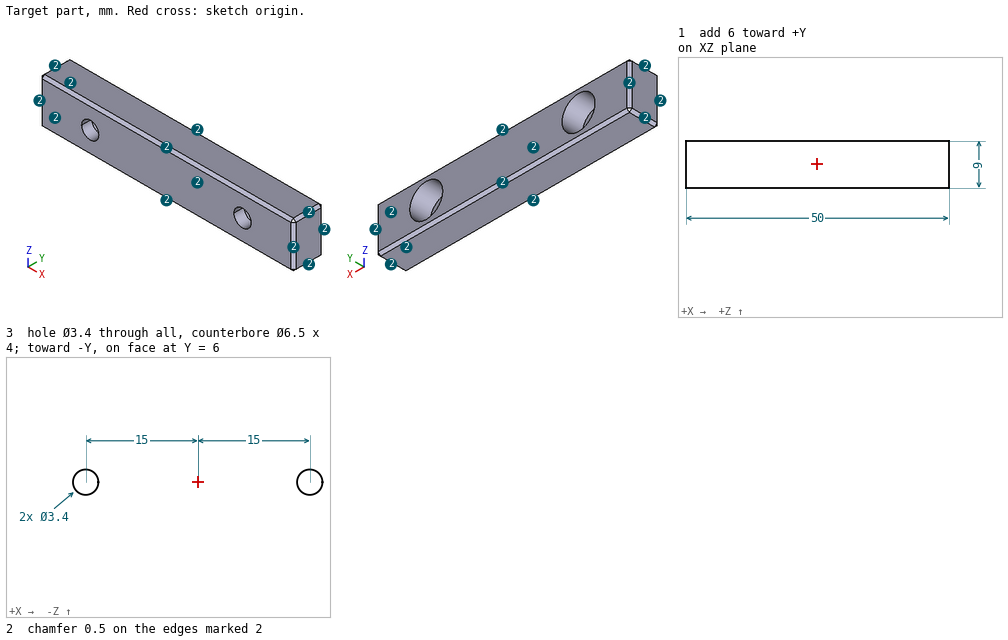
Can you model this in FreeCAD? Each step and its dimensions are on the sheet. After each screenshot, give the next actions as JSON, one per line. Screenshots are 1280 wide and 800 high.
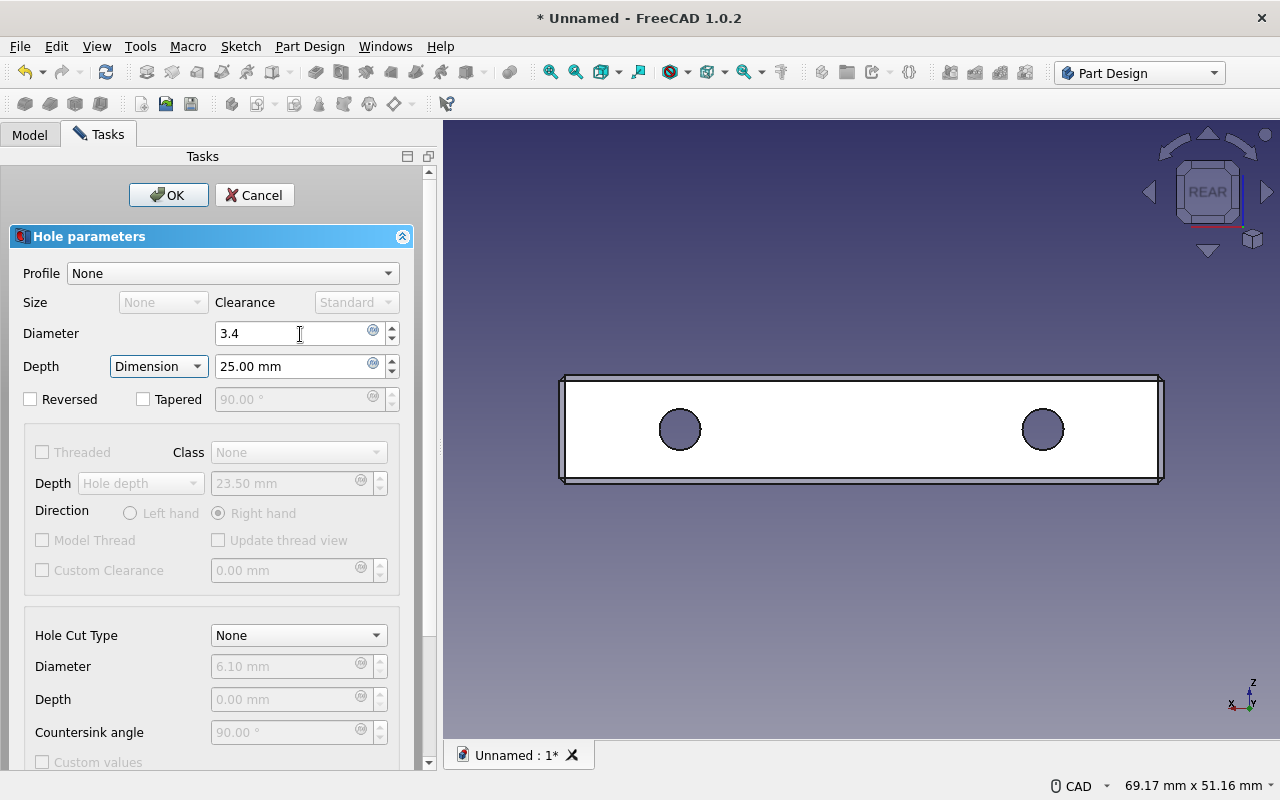
{"action": "left_click", "coordinate": [160, 366]}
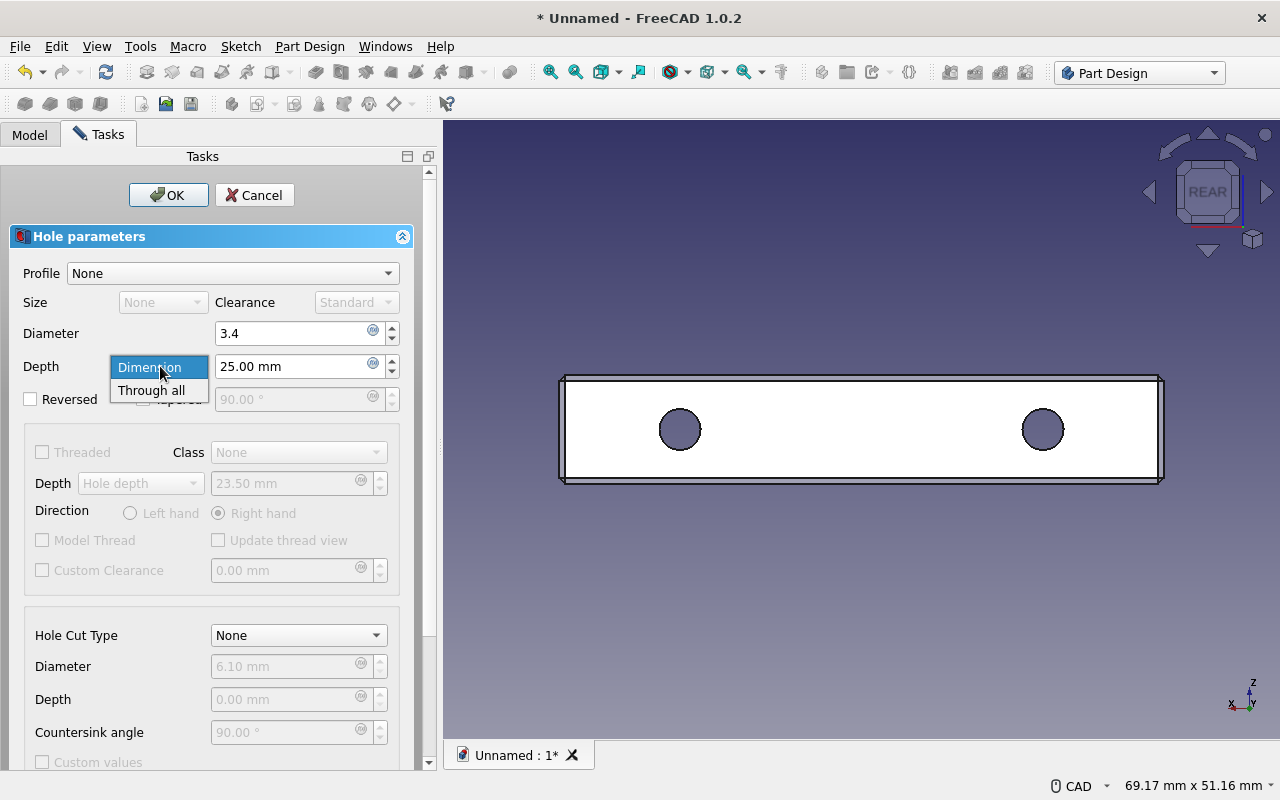
{"action": "left_click", "coordinate": [158, 390]}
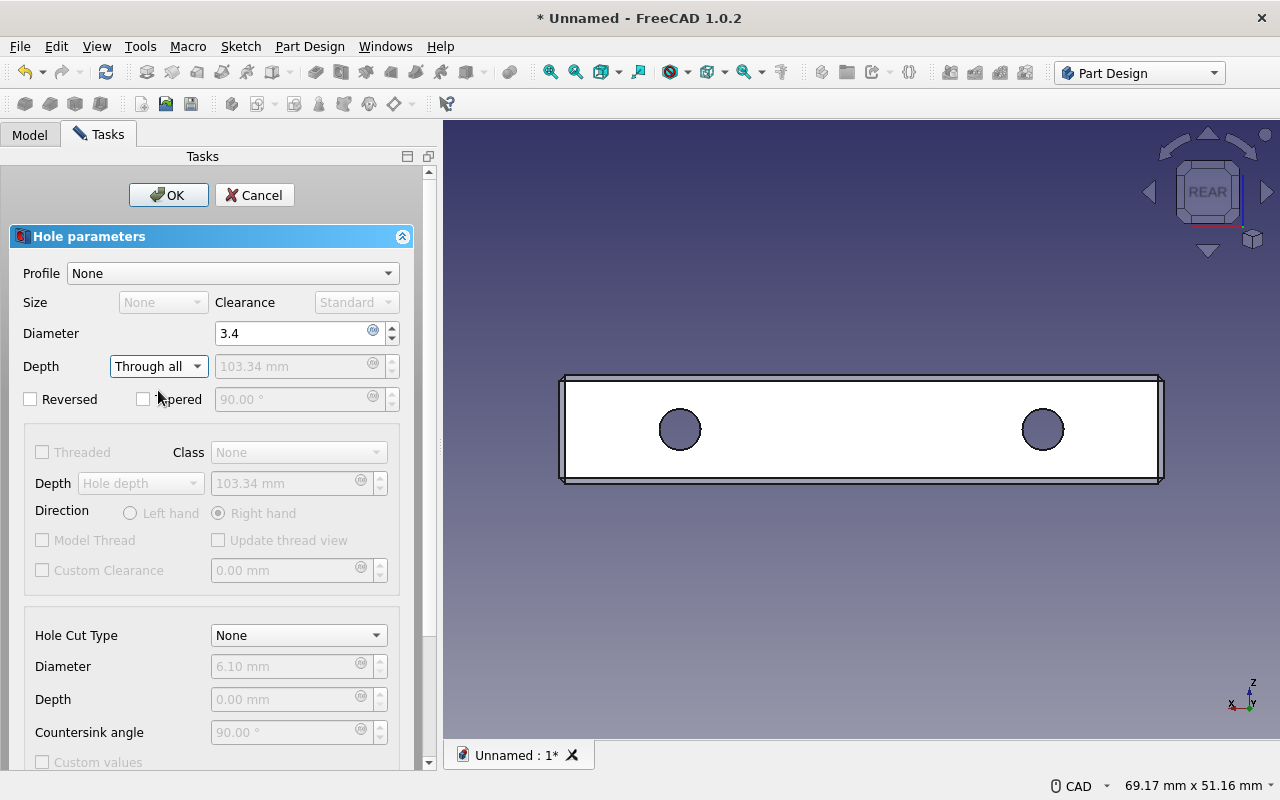
{"action": "left_click", "coordinate": [300, 636]}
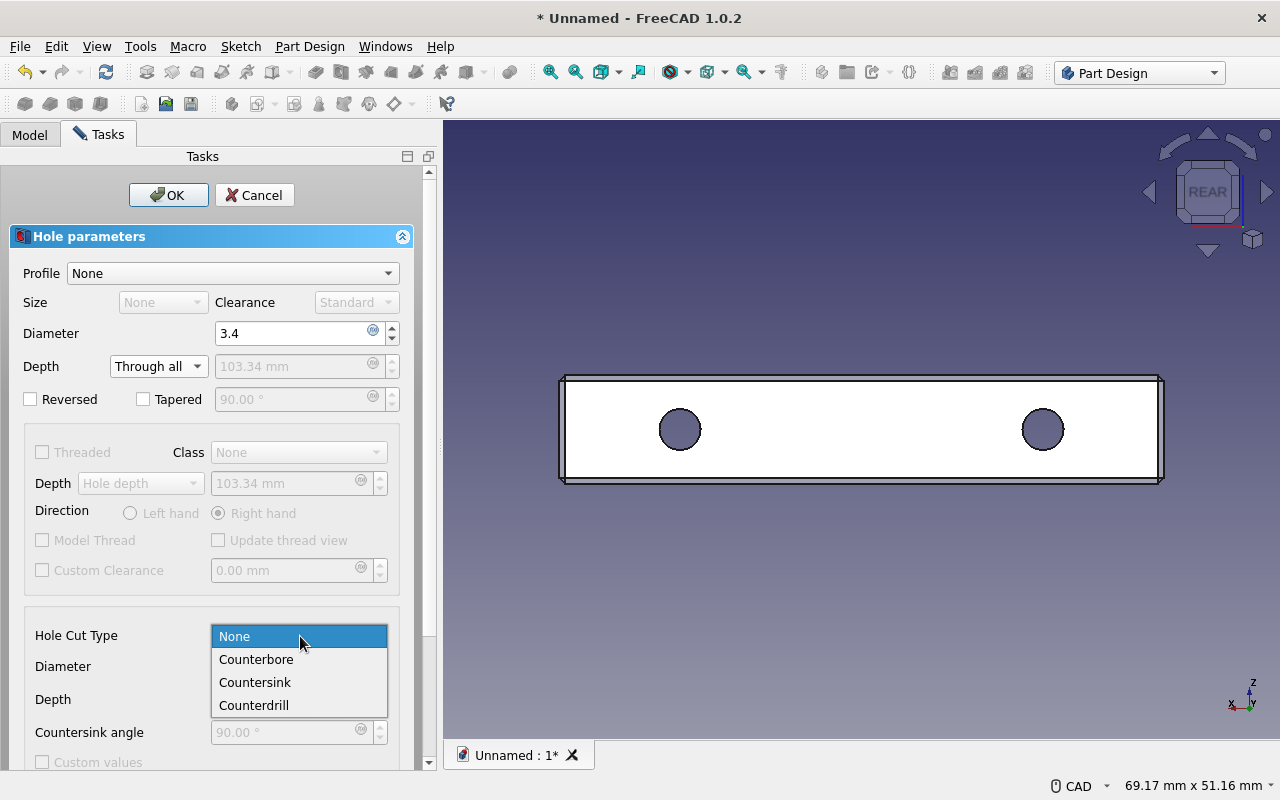
{"action": "left_click", "coordinate": [298, 660]}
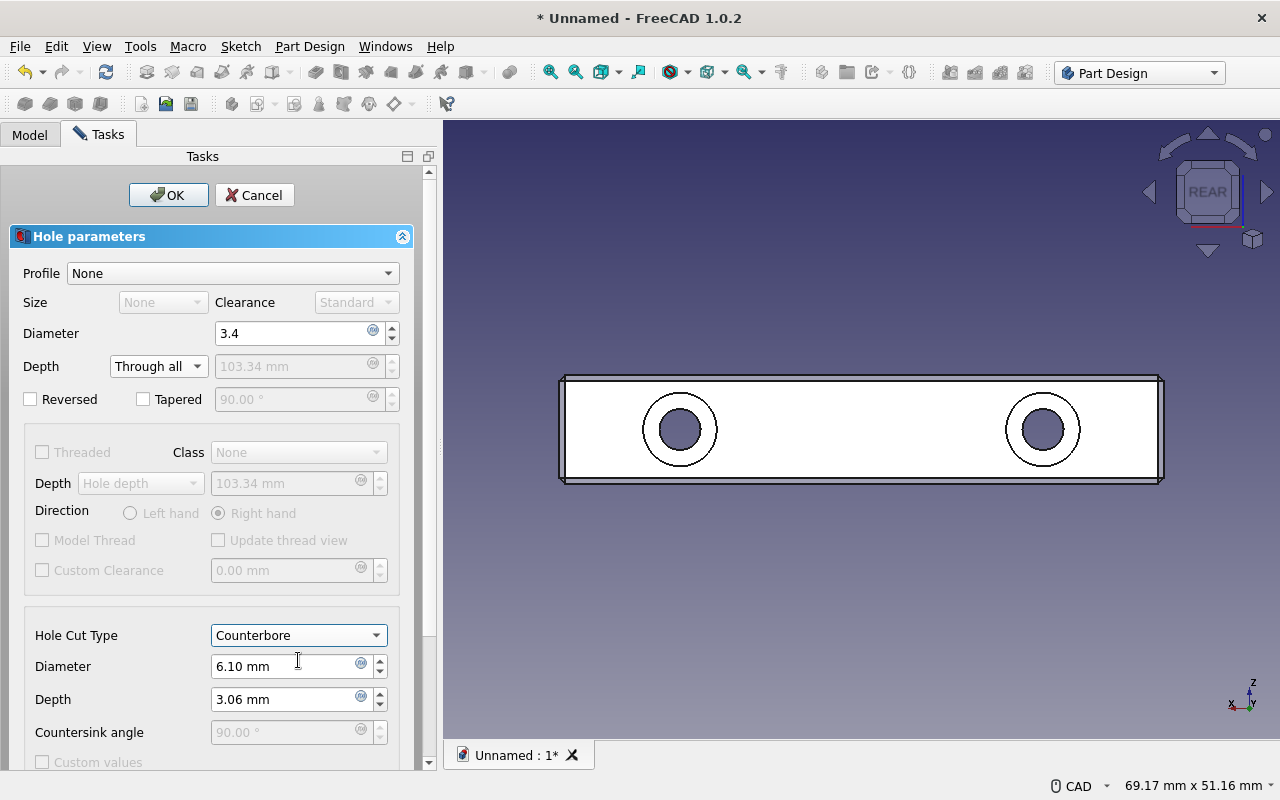
{"action": "triple_click", "coordinate": [292, 666]}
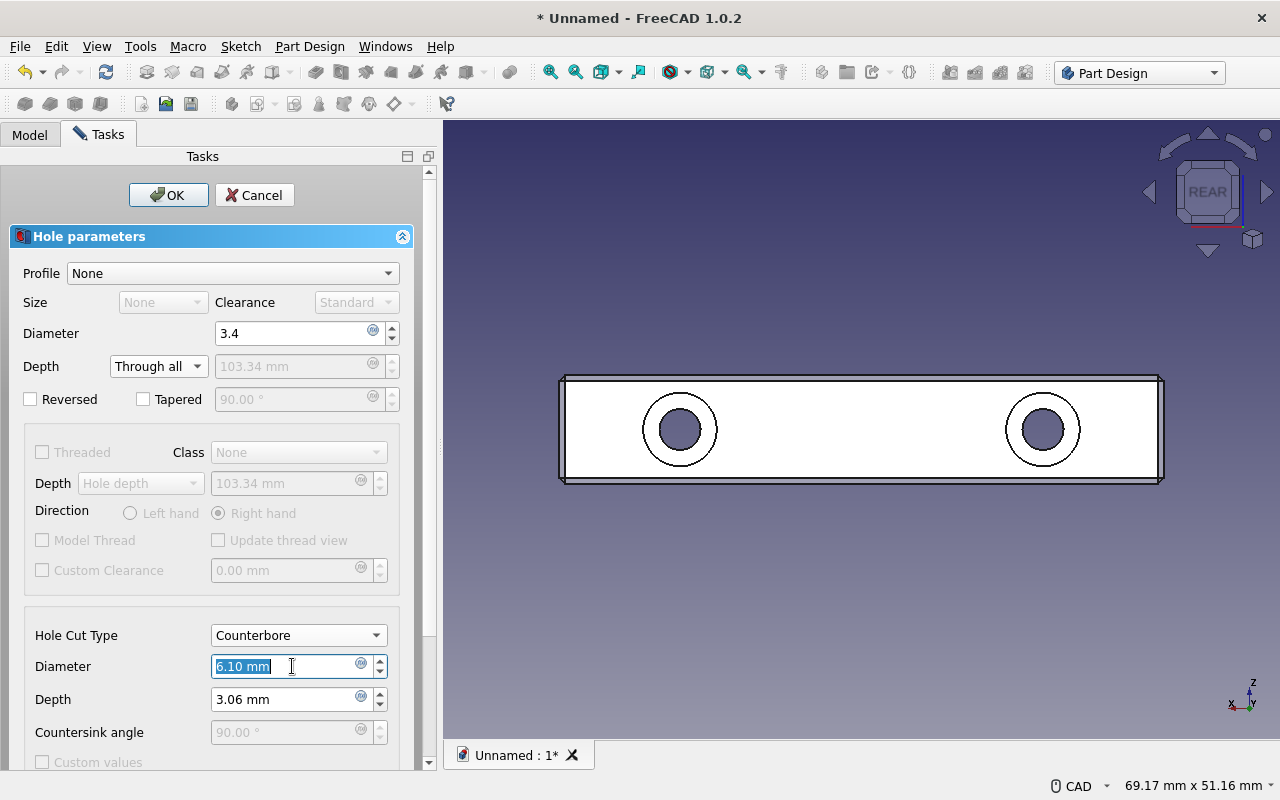
{"action": "type", "text": "6.5"}
{"action": "key", "text": "Tab"}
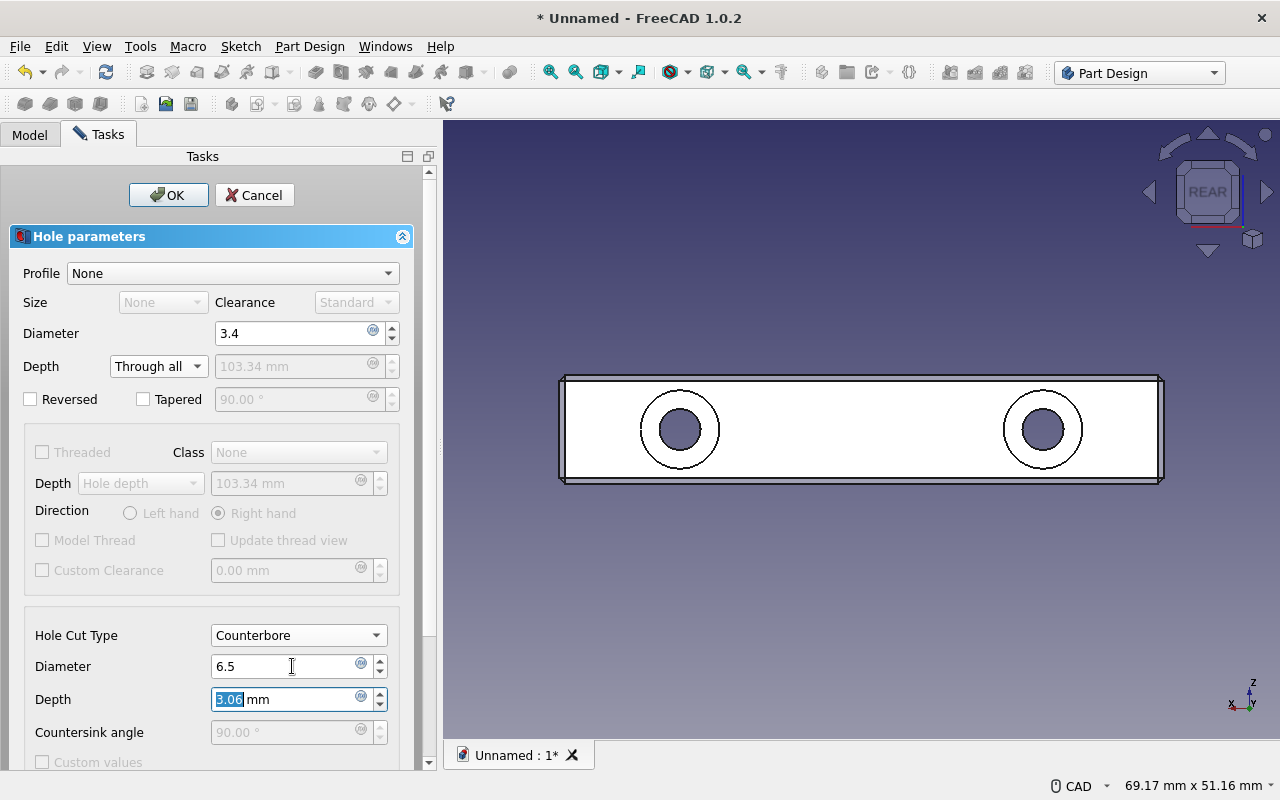
{"action": "type", "text": "4"}
{"action": "key", "text": "Tab"}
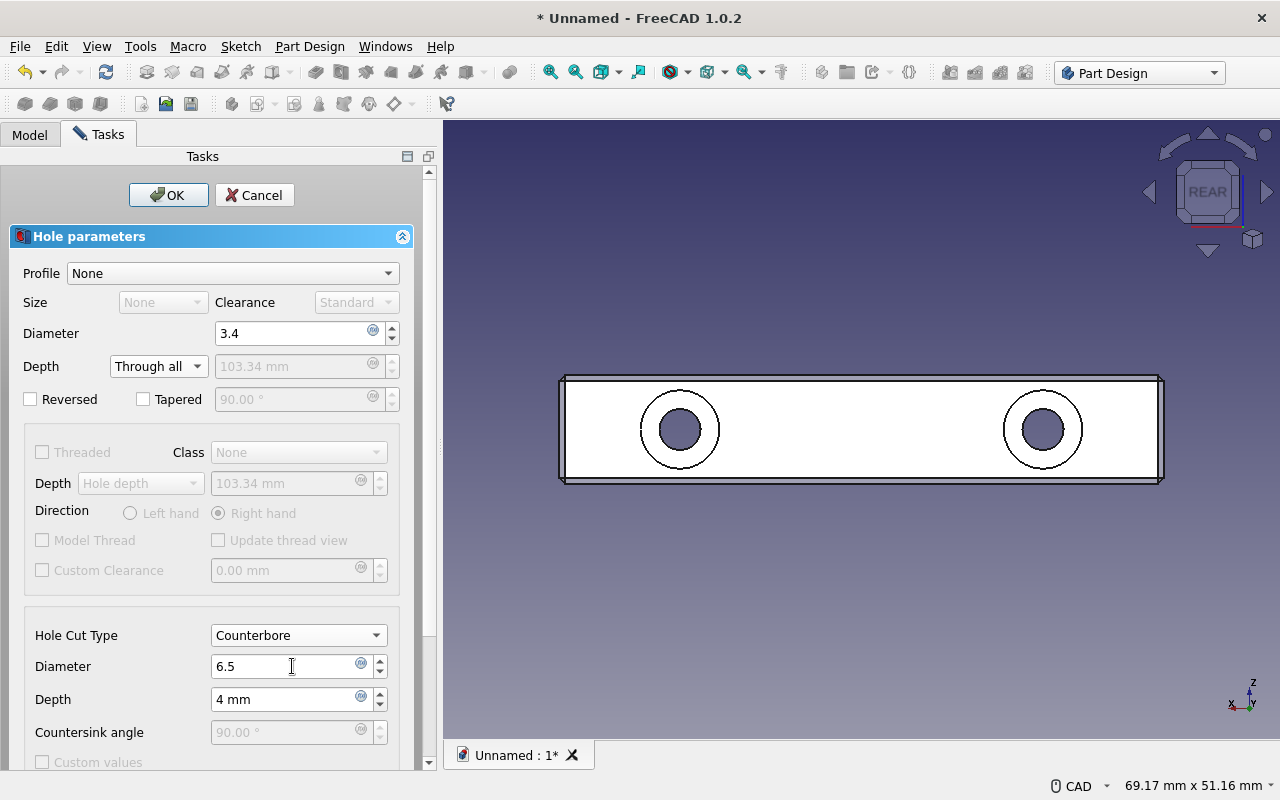
{"action": "left_click", "coordinate": [169, 195]}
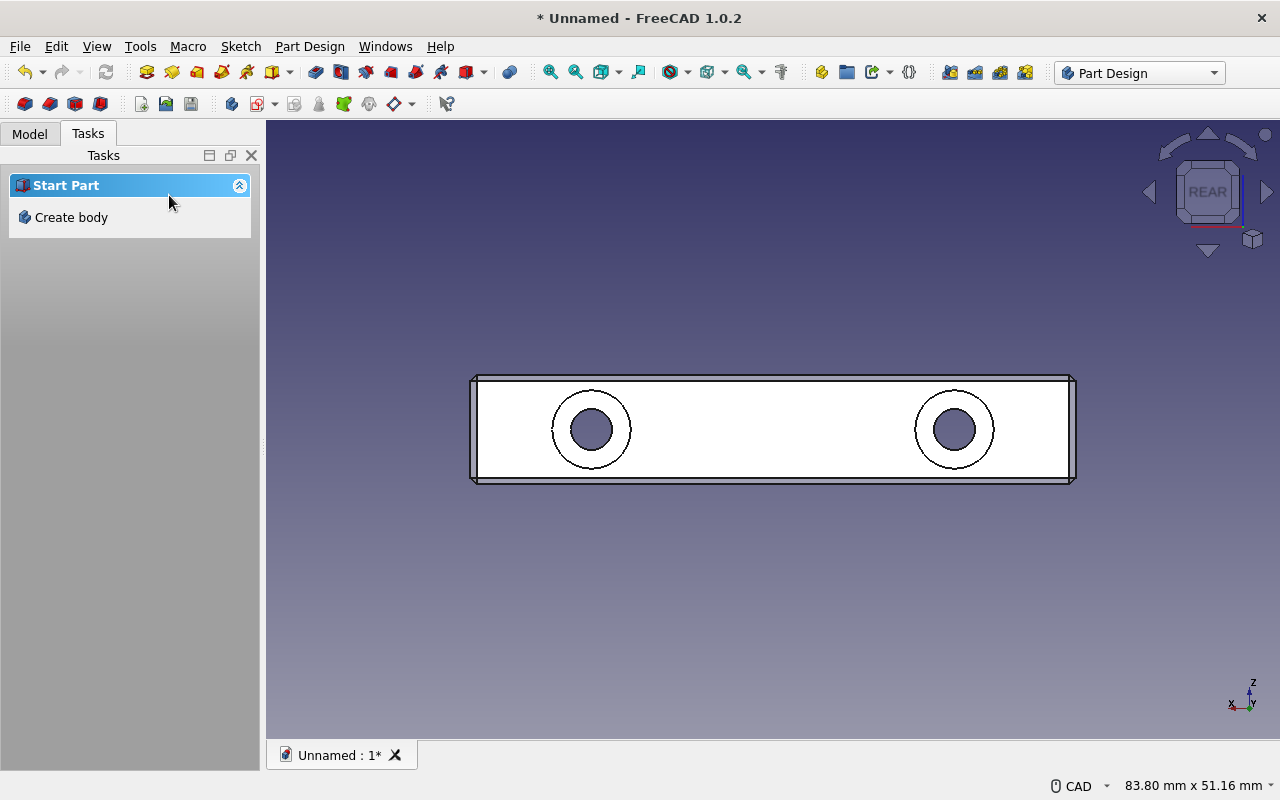
{"action": "key", "text": "0"}